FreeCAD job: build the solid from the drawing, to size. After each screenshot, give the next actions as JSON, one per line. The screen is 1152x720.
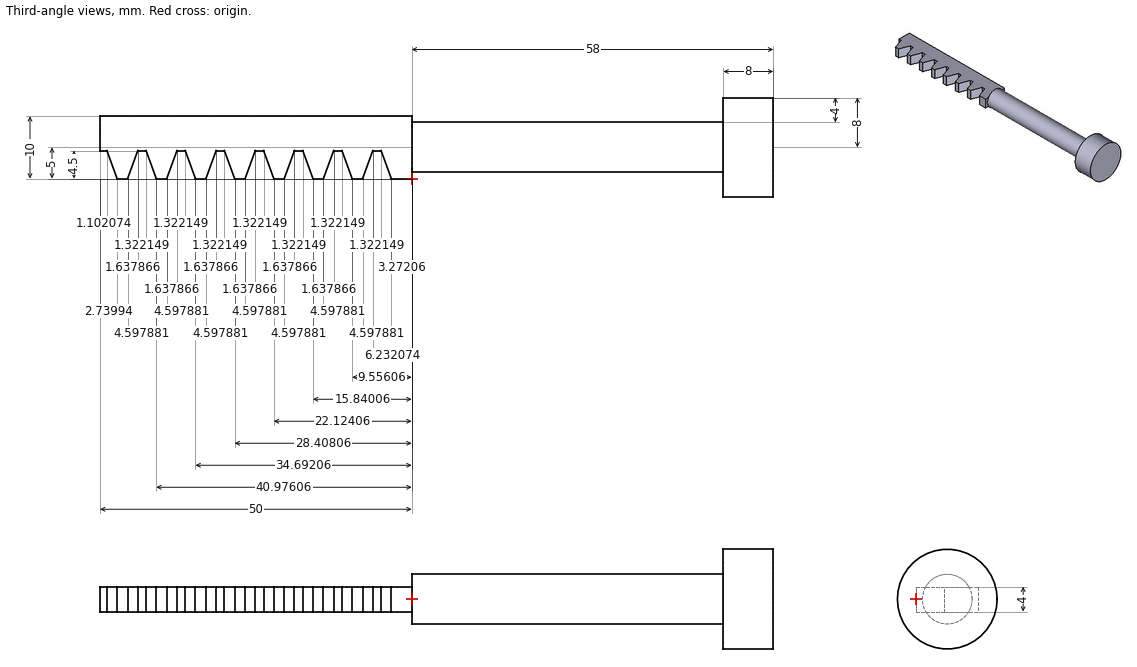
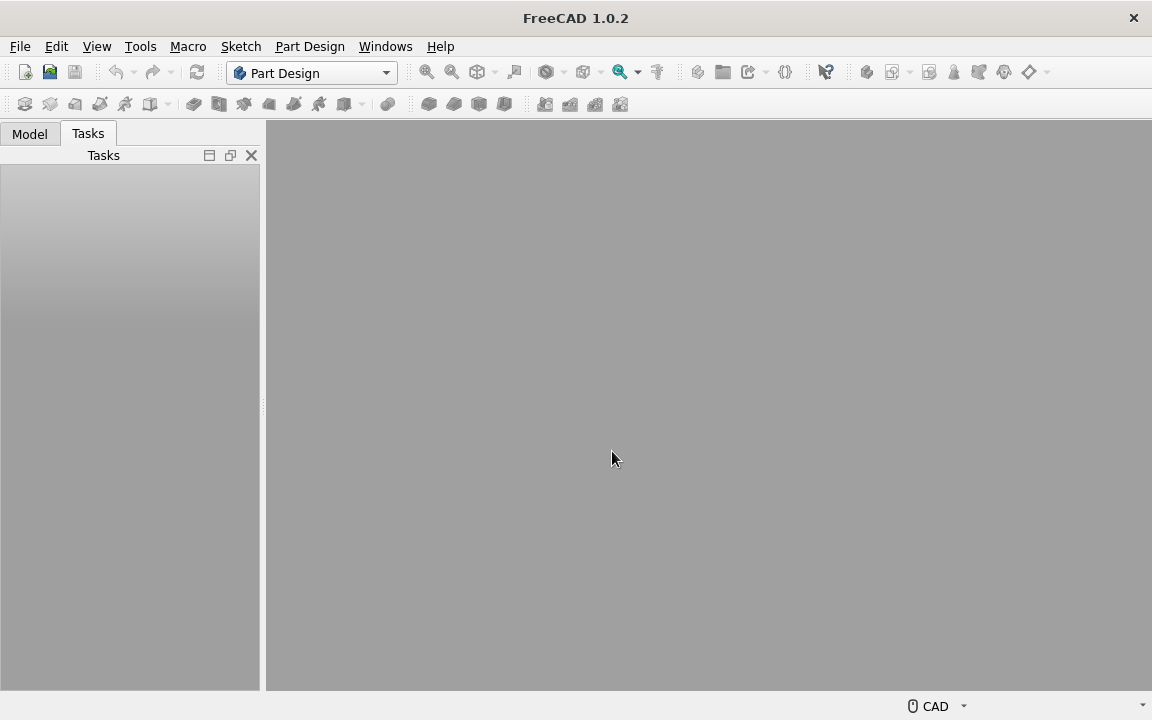
{"action": "left_click", "coordinate": [25, 72]}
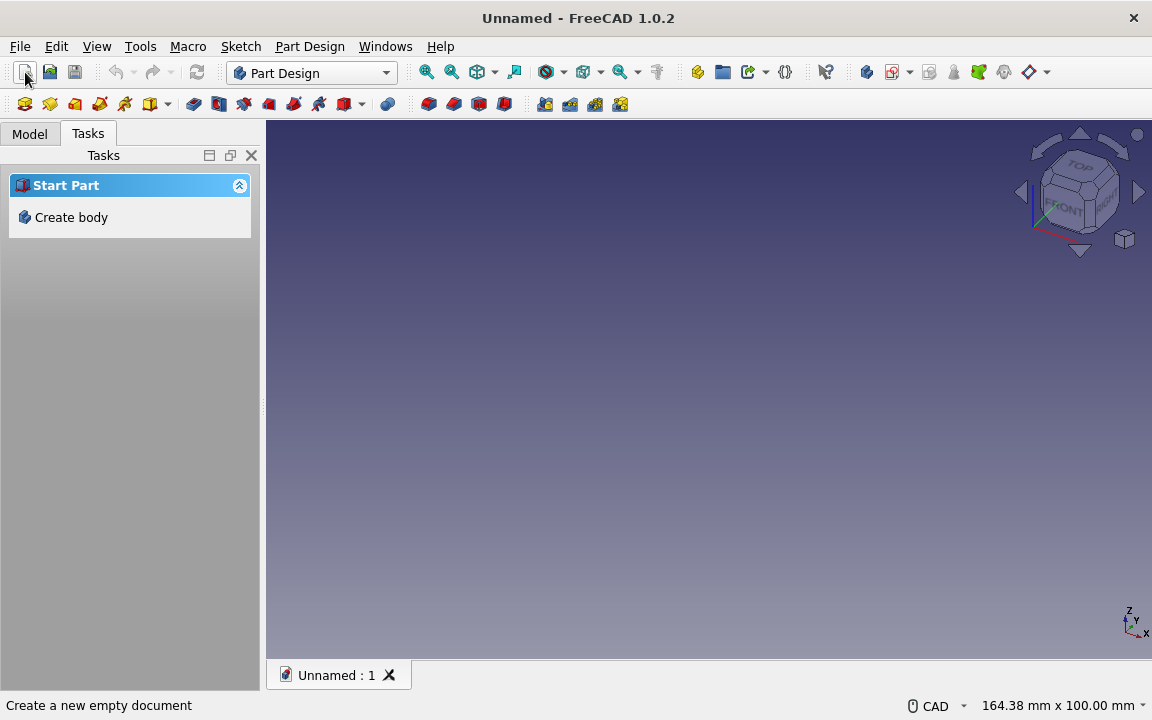
{"action": "left_click", "coordinate": [867, 72]}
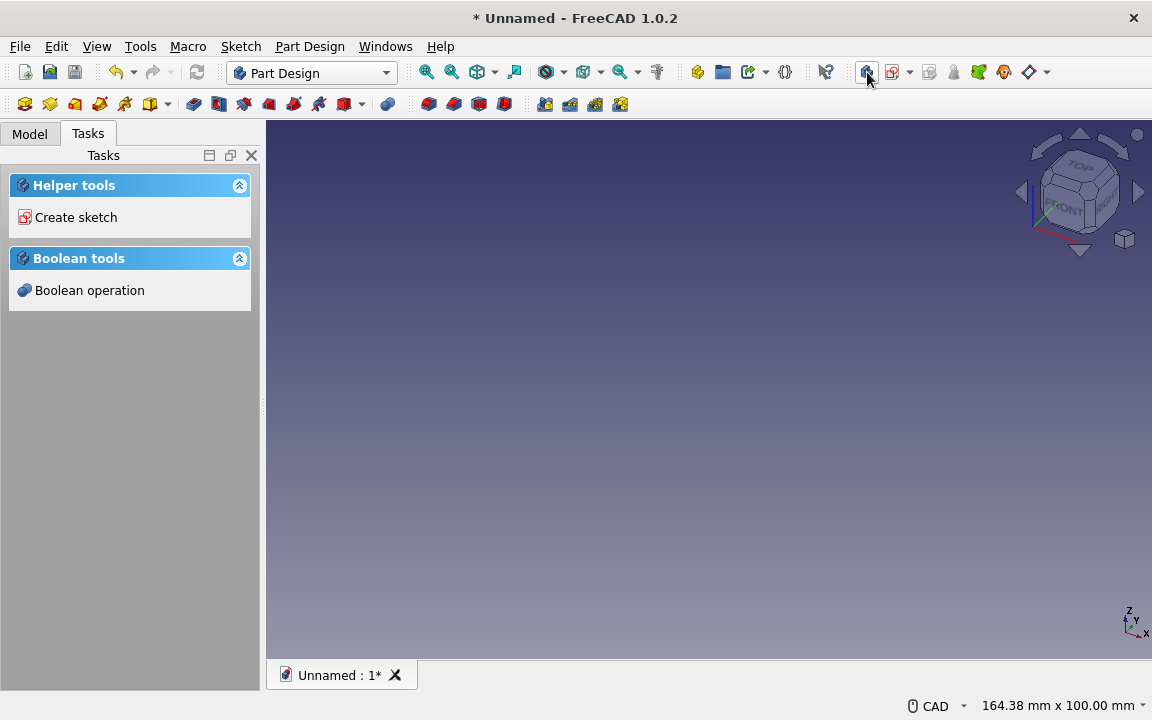
{"action": "left_click", "coordinate": [30, 134]}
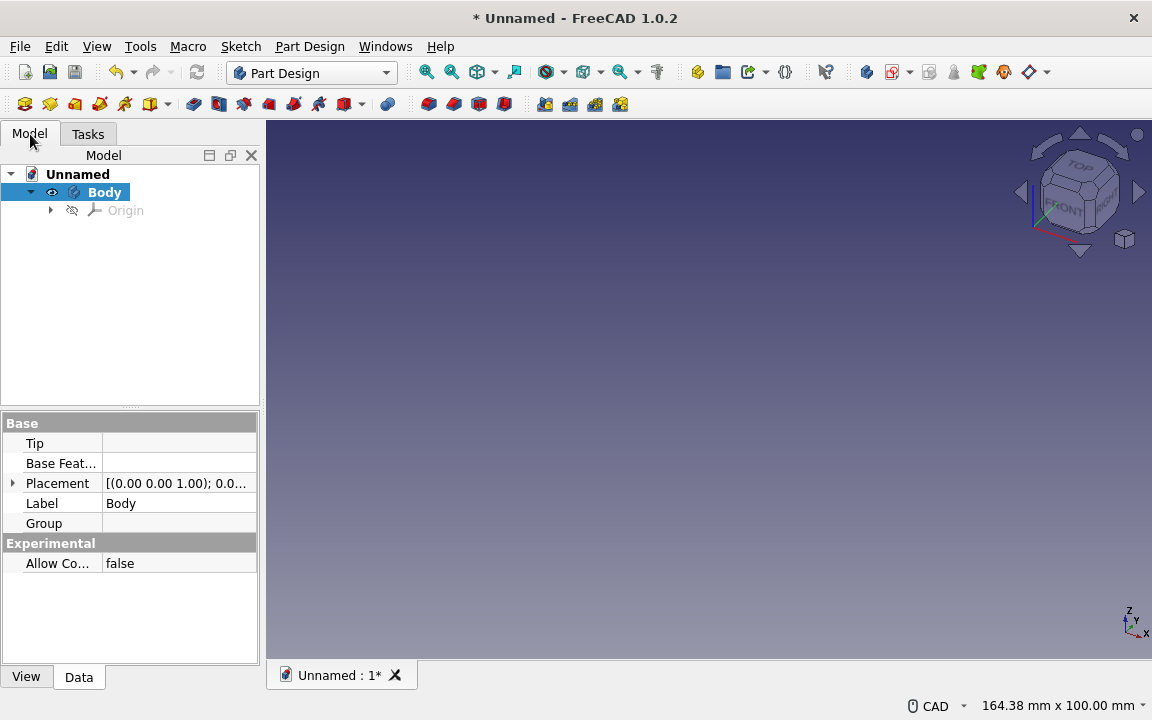
{"action": "left_click", "coordinate": [51, 210]}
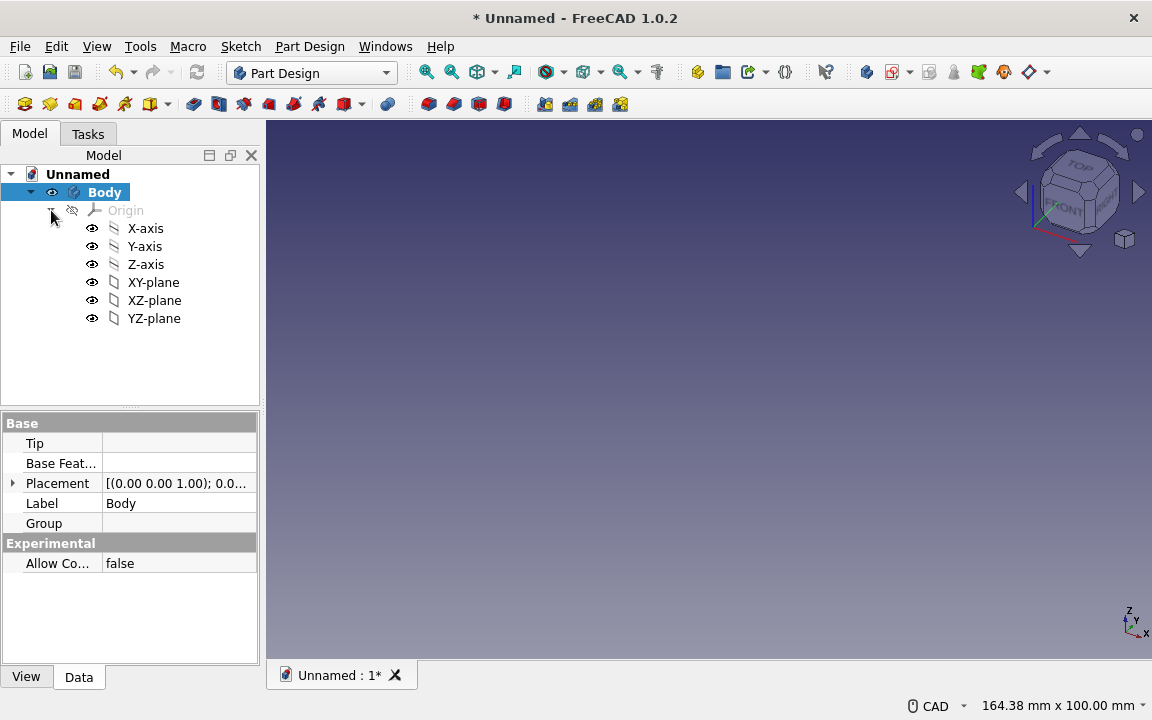
{"action": "left_click", "coordinate": [137, 282]}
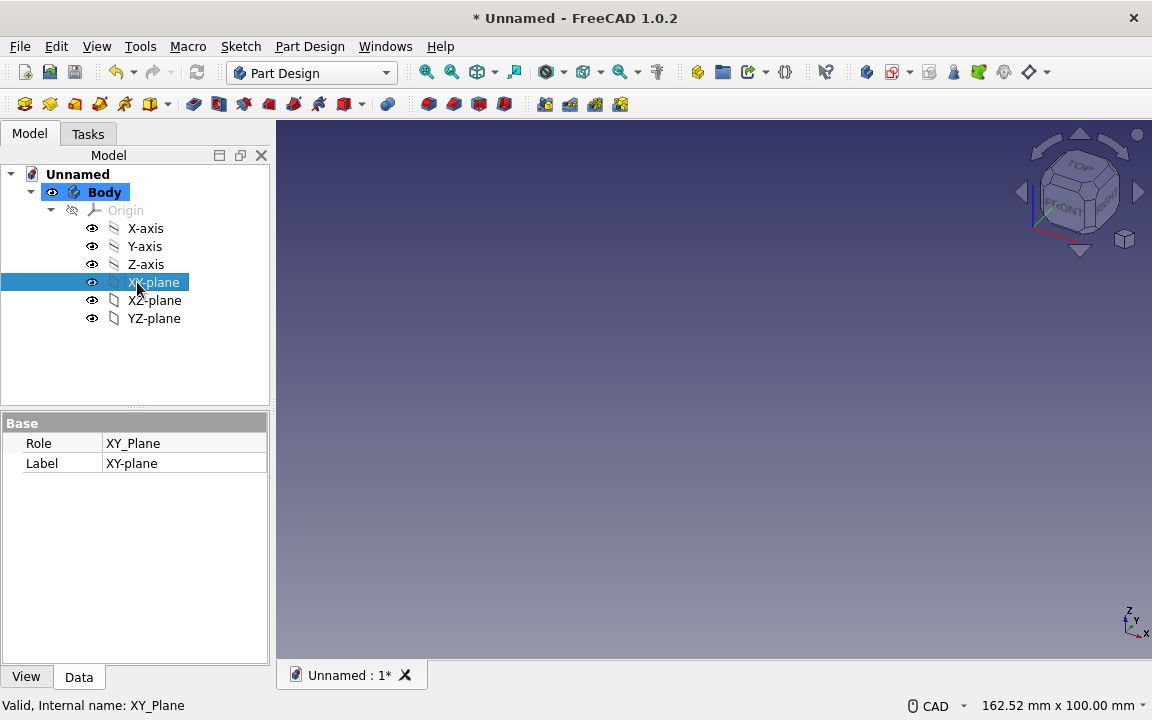
{"action": "left_click", "coordinate": [1028, 72]}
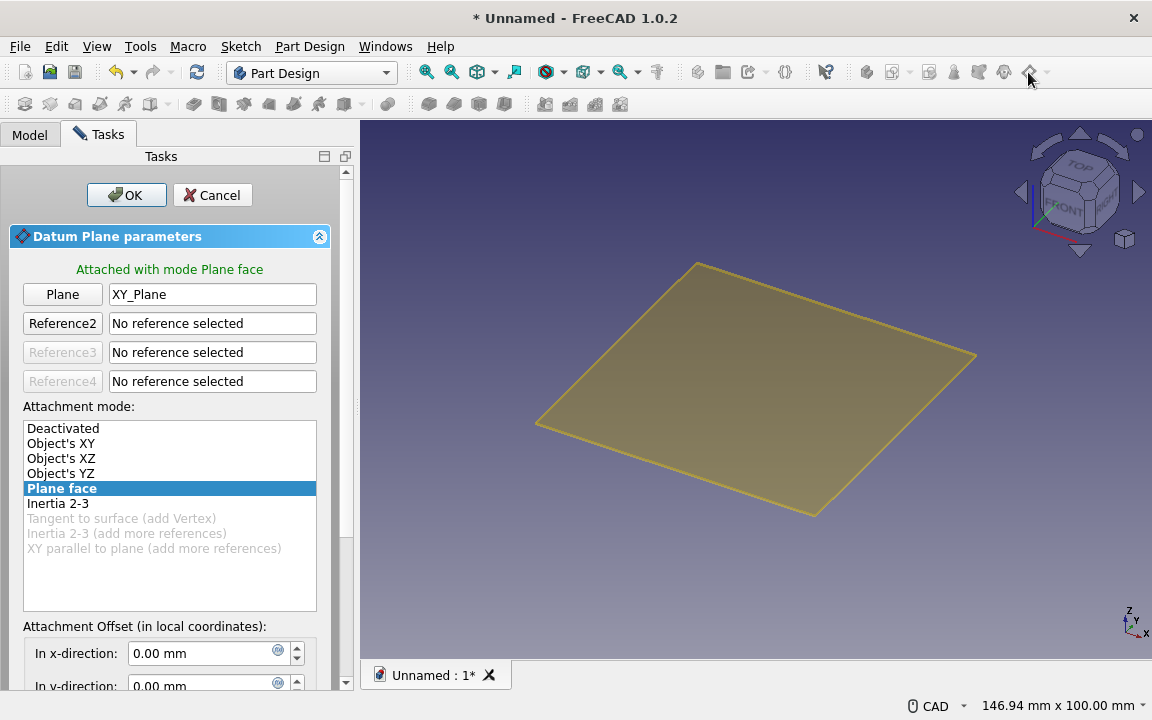
{"action": "scroll", "coordinate": [346, 428], "scroll_direction": "down", "scroll_amount": 2}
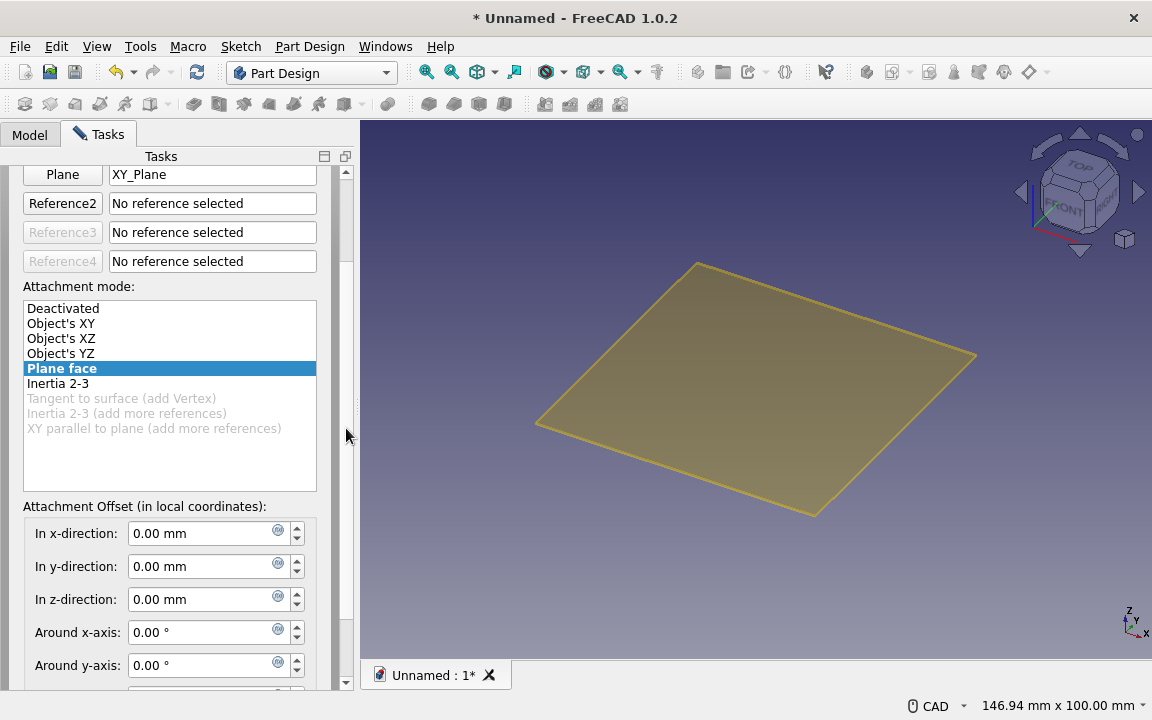
{"action": "triple_click", "coordinate": [210, 600]}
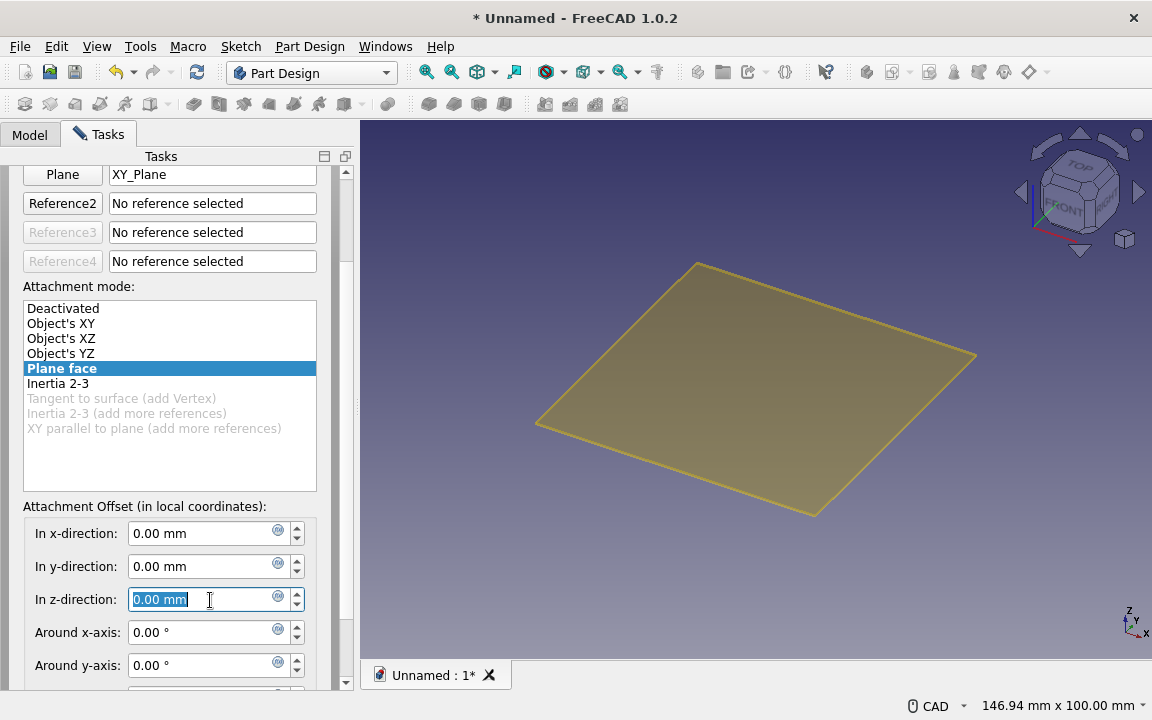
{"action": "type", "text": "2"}
{"action": "key", "text": "Tab"}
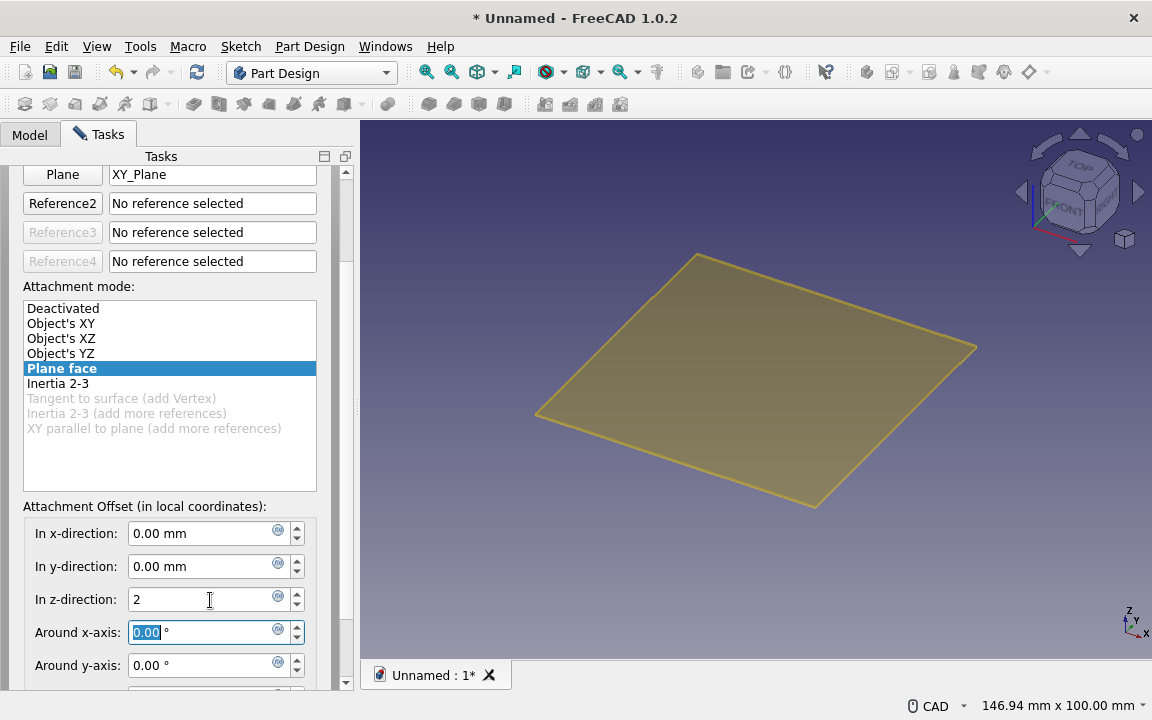
{"action": "scroll", "coordinate": [346, 428], "scroll_direction": "up", "scroll_amount": 3}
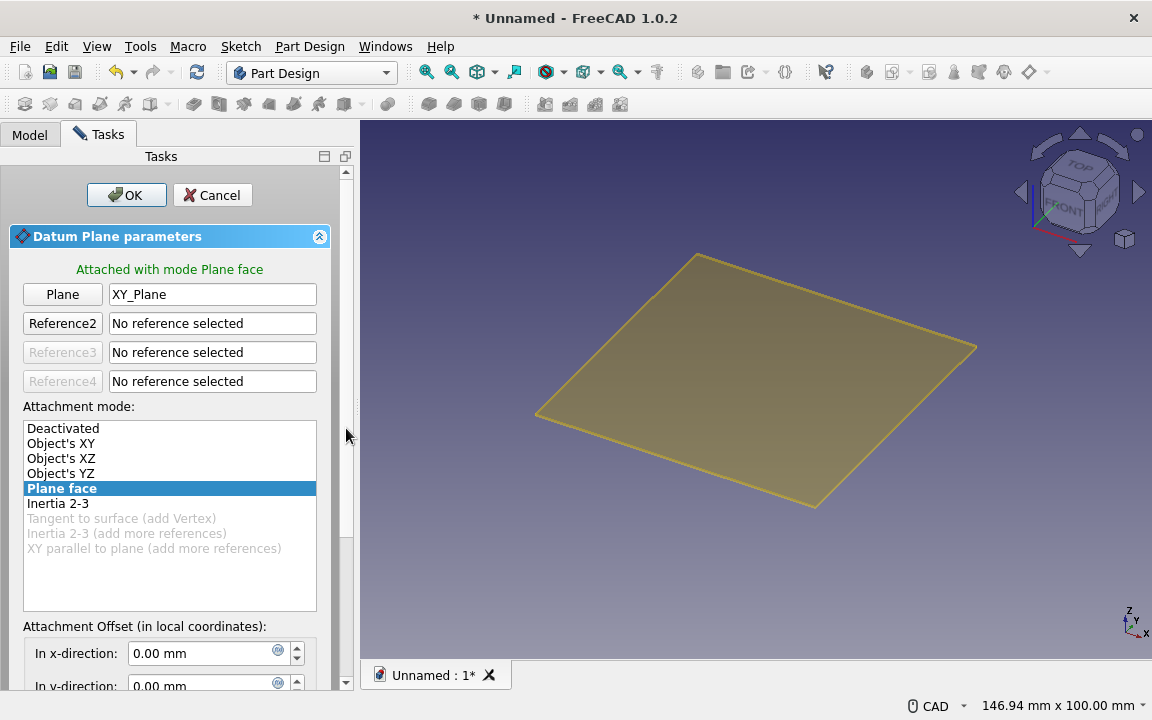
{"action": "left_click", "coordinate": [127, 195]}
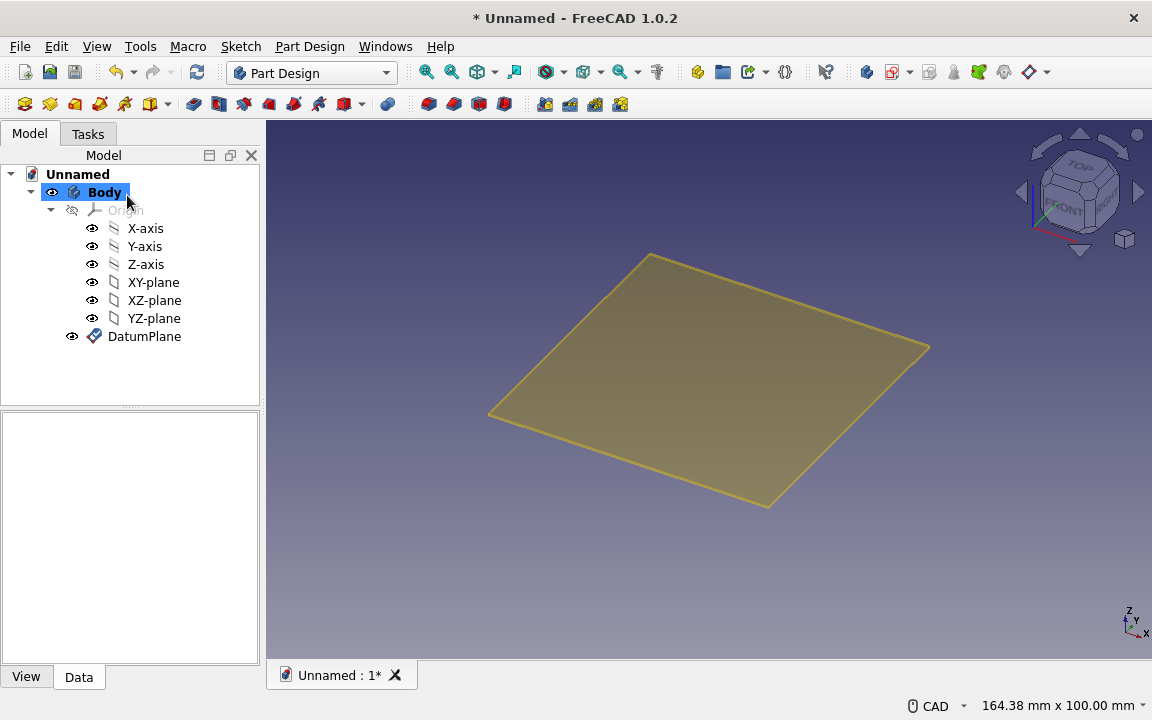
{"action": "left_click", "coordinate": [117, 336]}